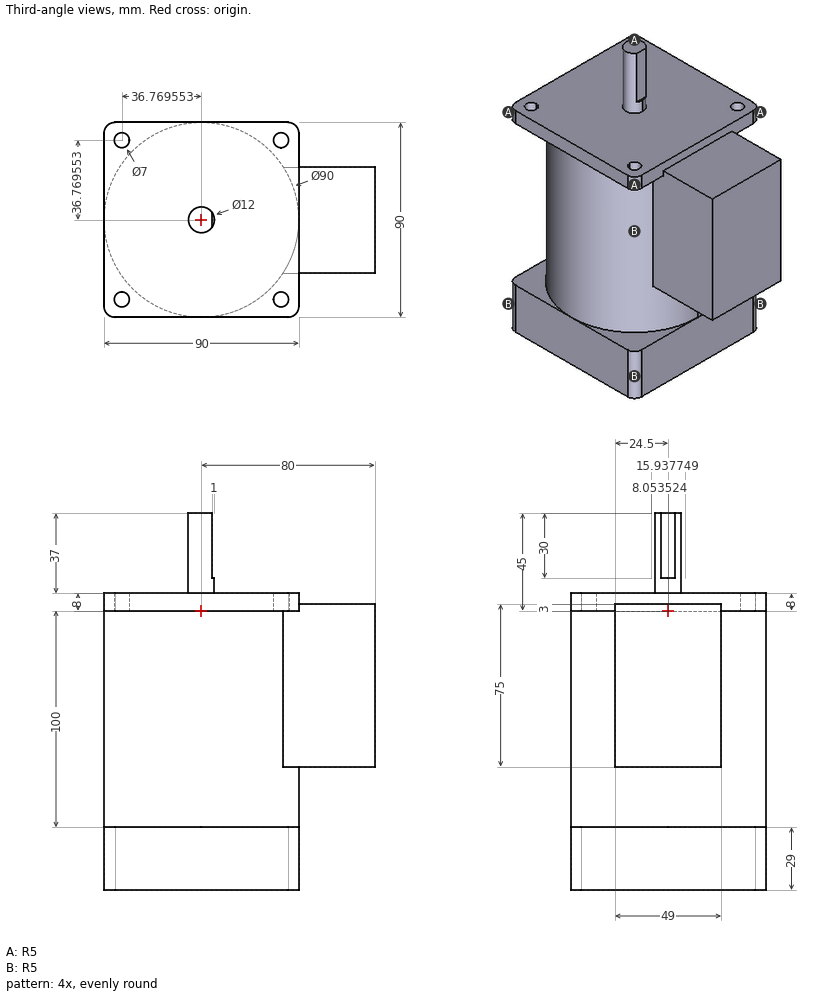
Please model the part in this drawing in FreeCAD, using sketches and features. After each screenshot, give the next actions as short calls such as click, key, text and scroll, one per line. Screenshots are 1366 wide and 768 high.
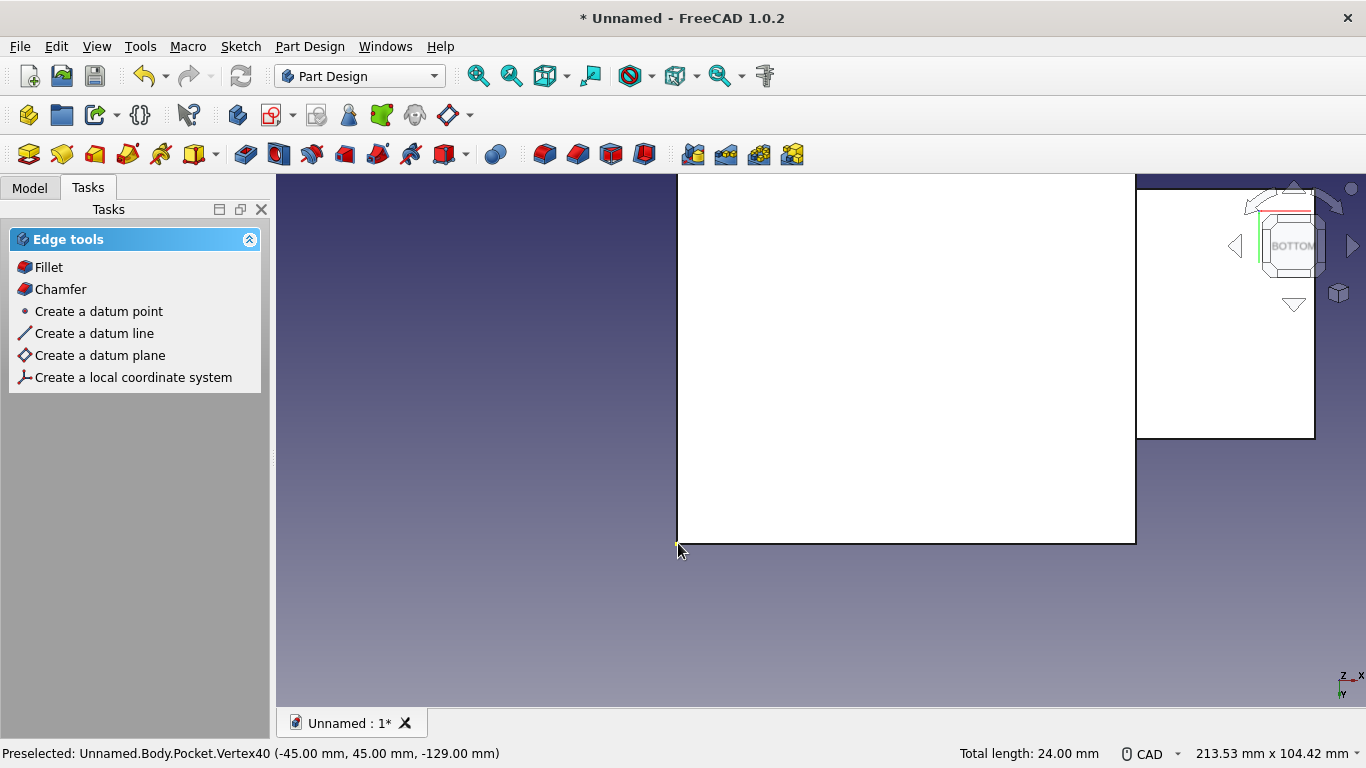
key(v)
key(f)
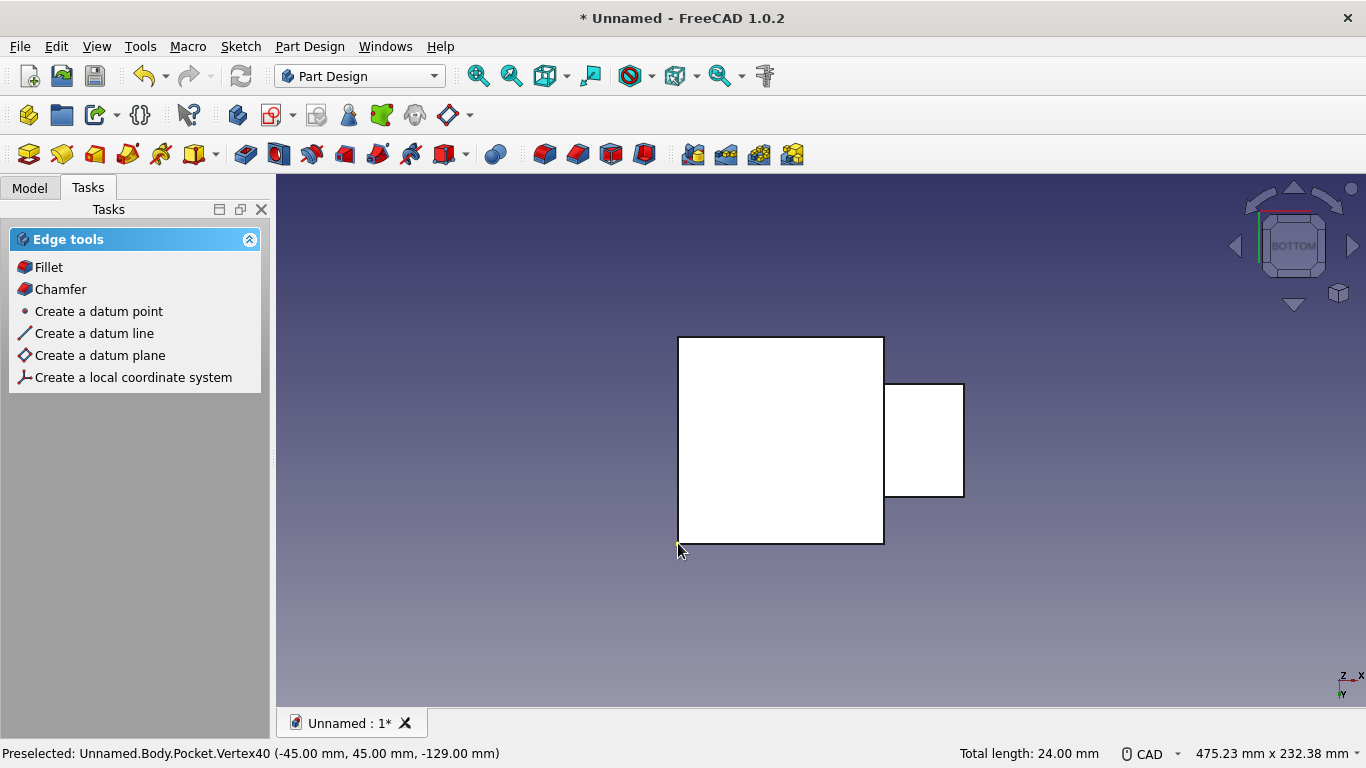
key(4)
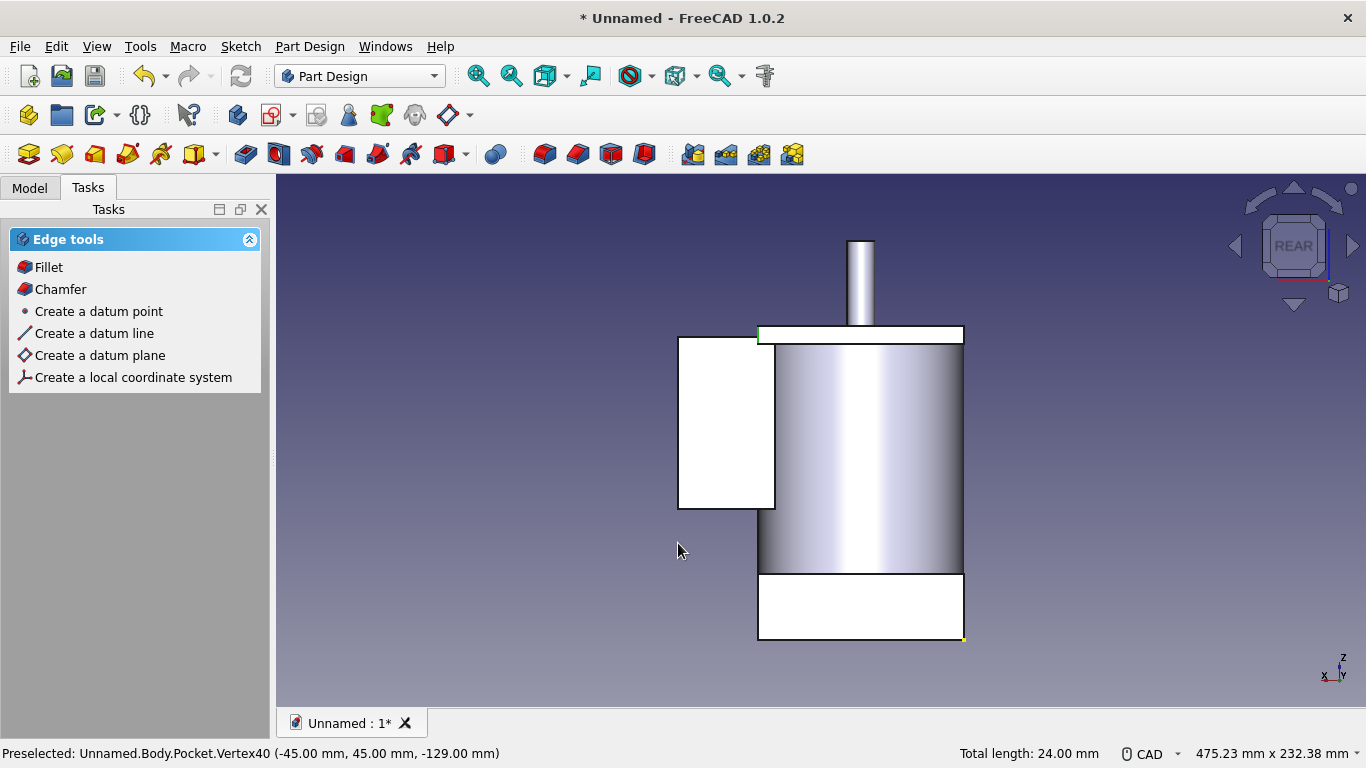
click(964, 334, ctrl)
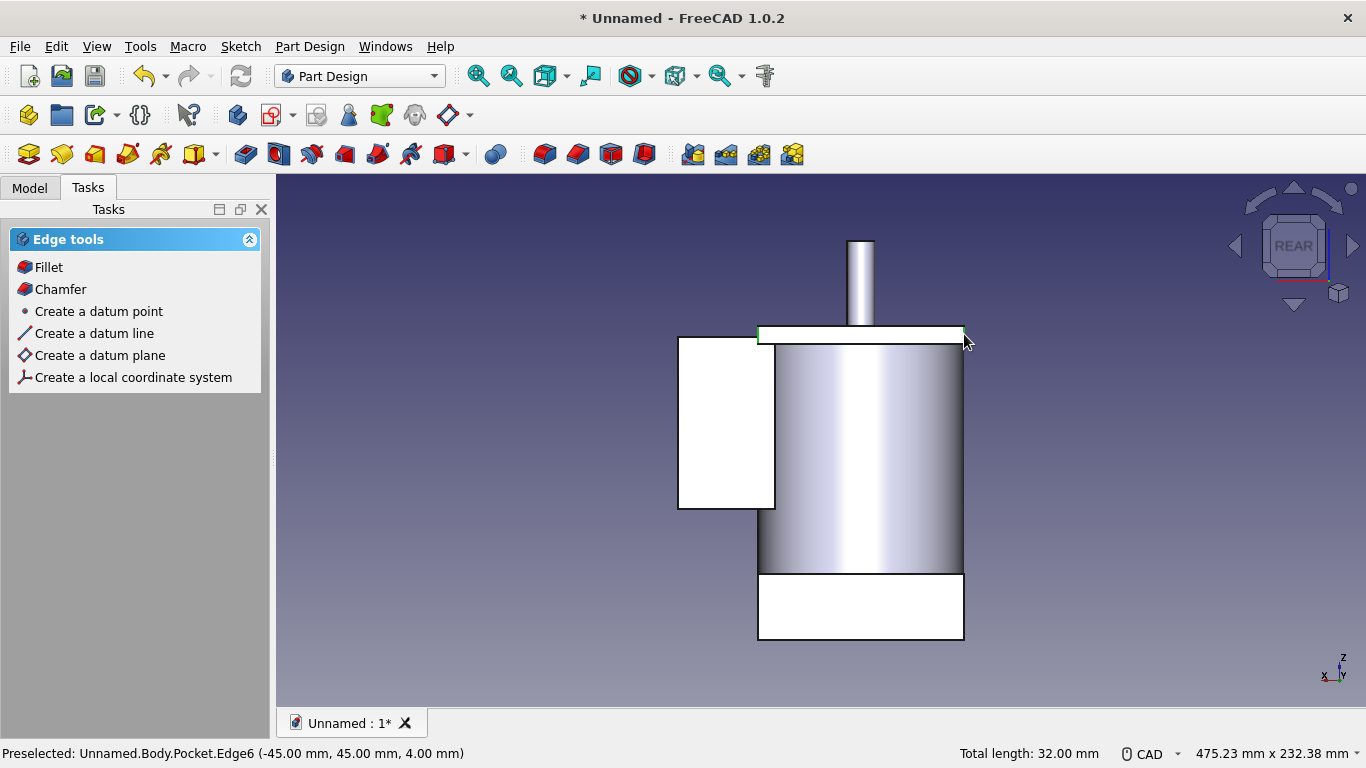
click(545, 154)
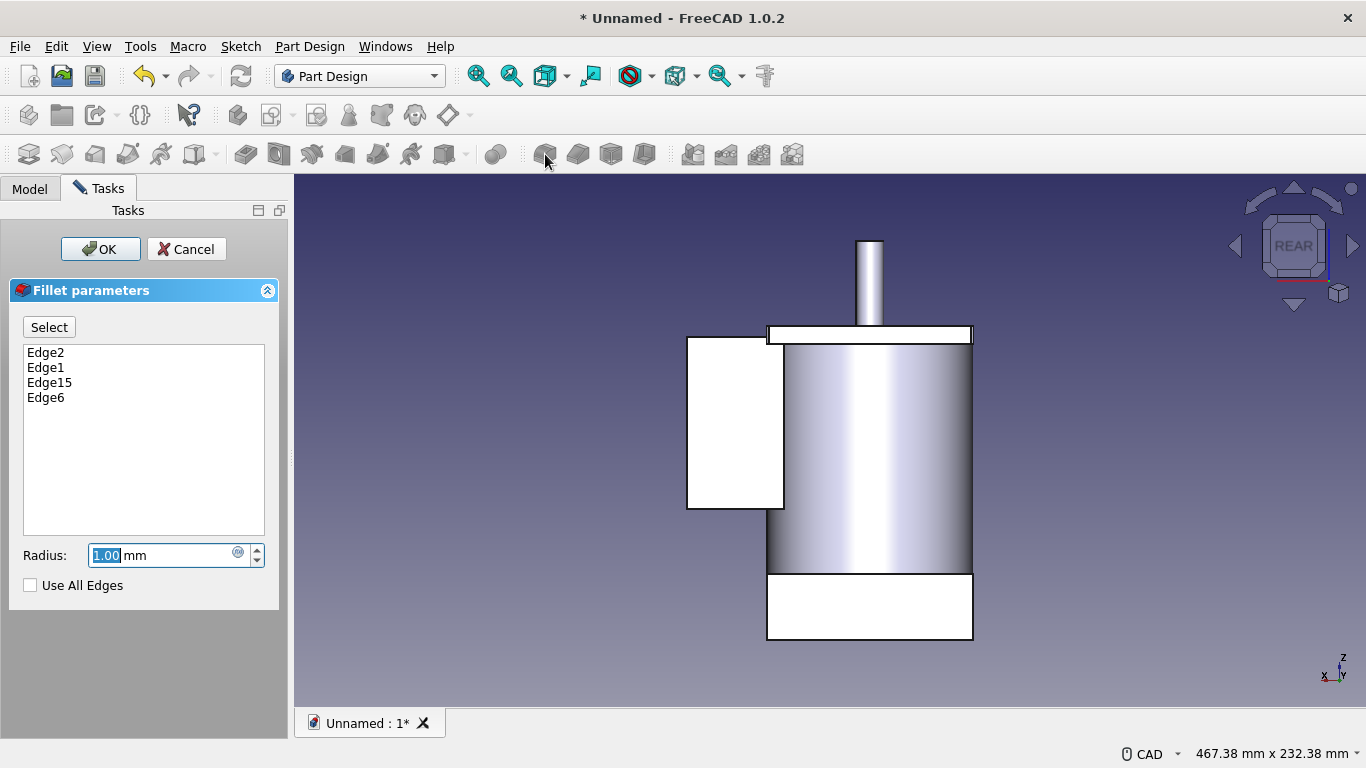
text(5)
key(Tab)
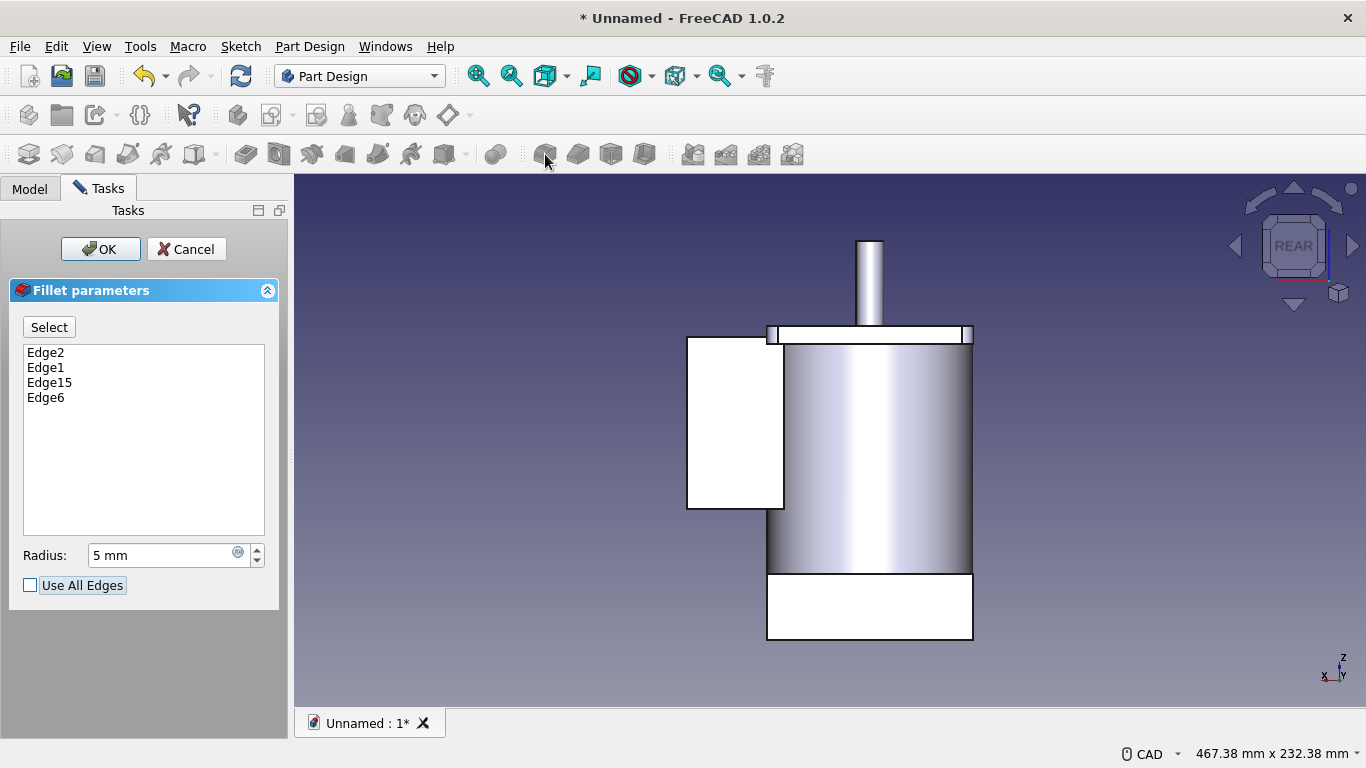
click(101, 249)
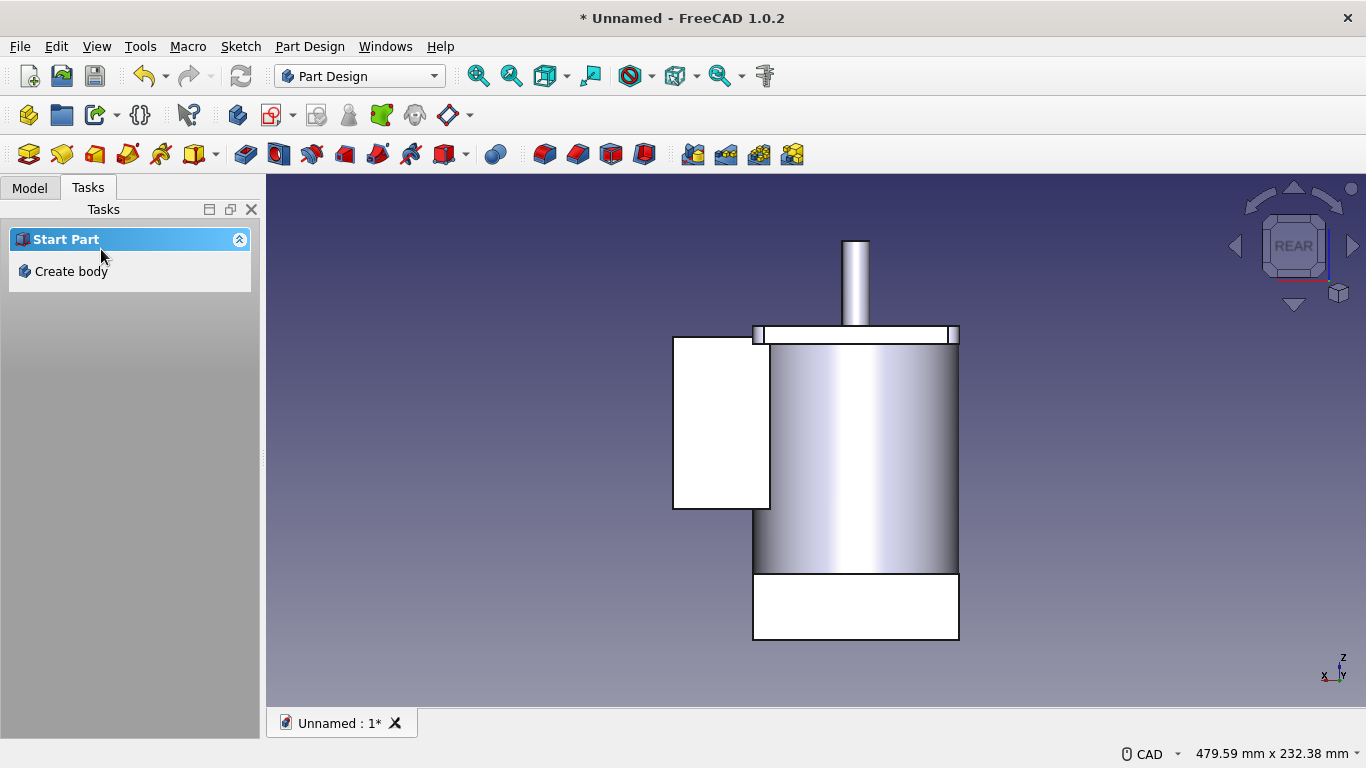
click(753, 606)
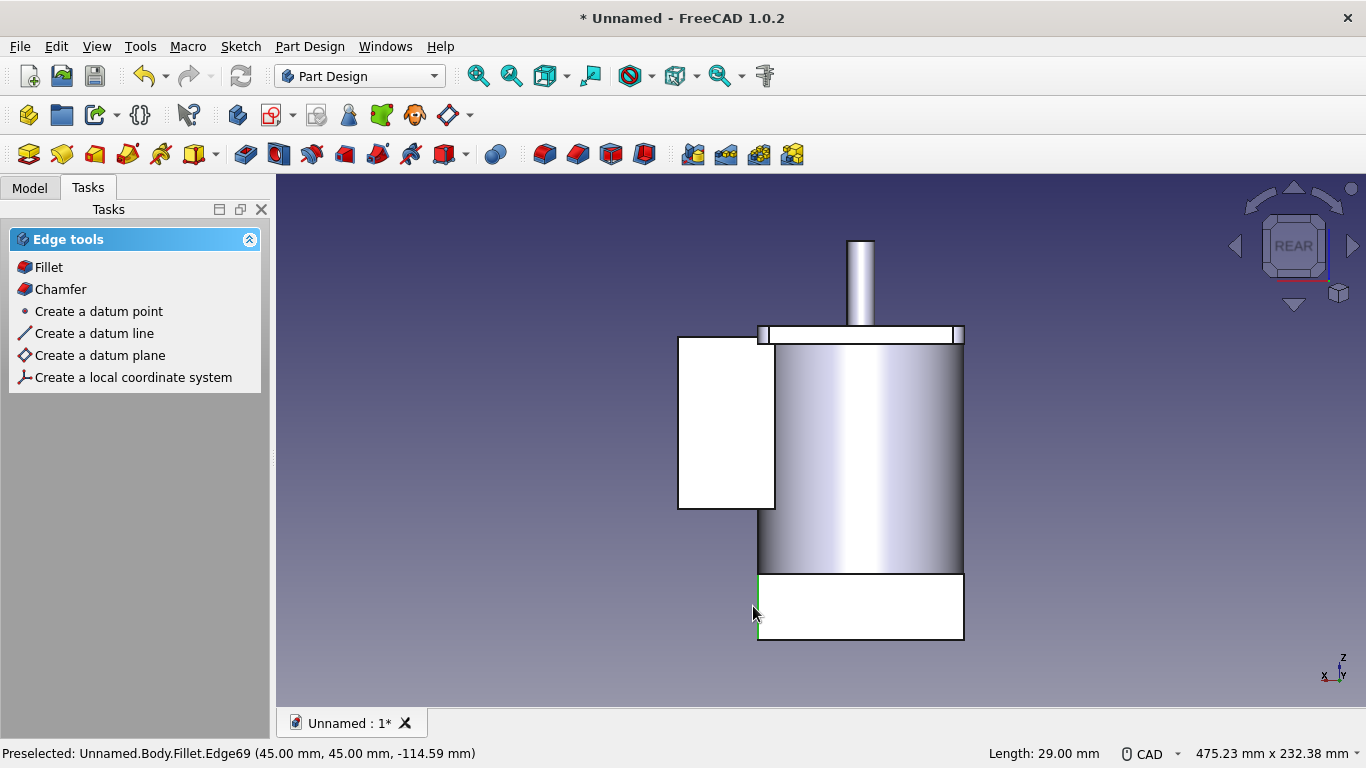
click(964, 606, ctrl)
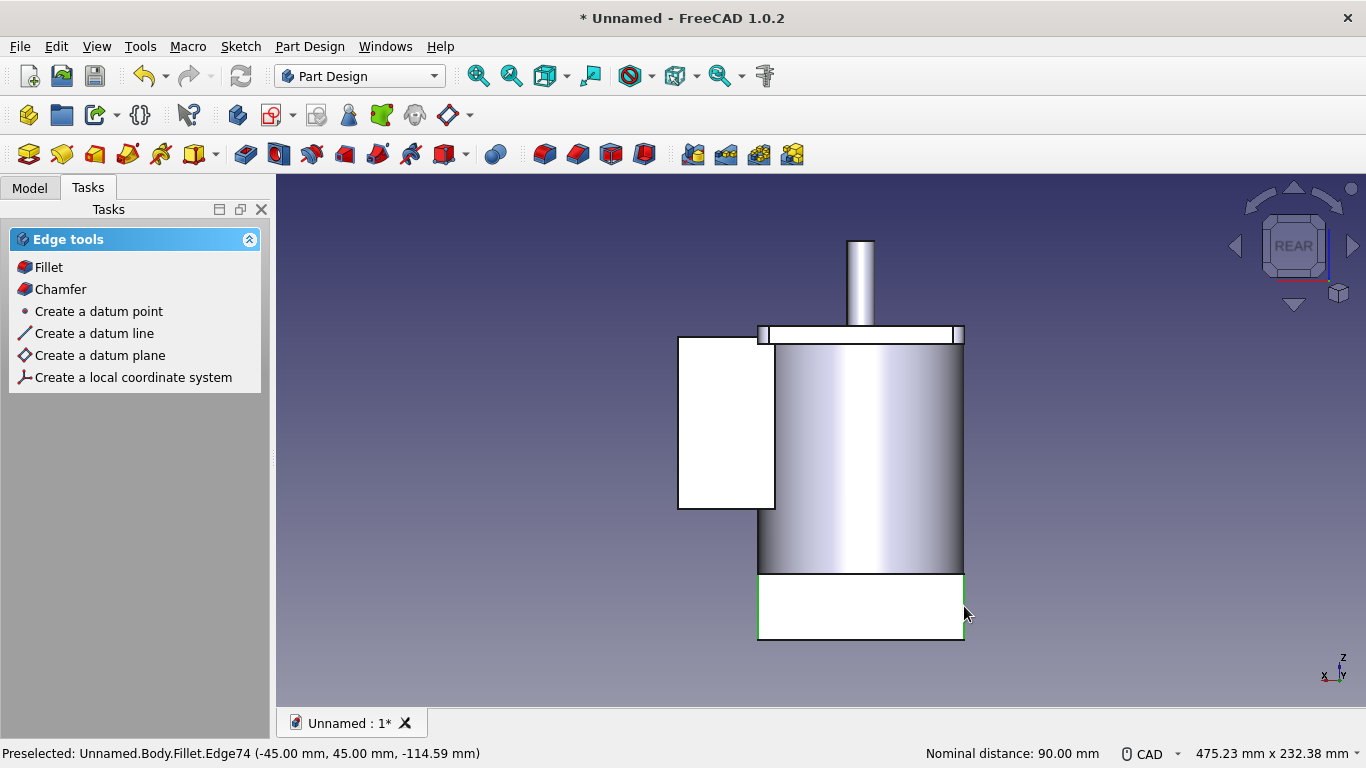
key(0)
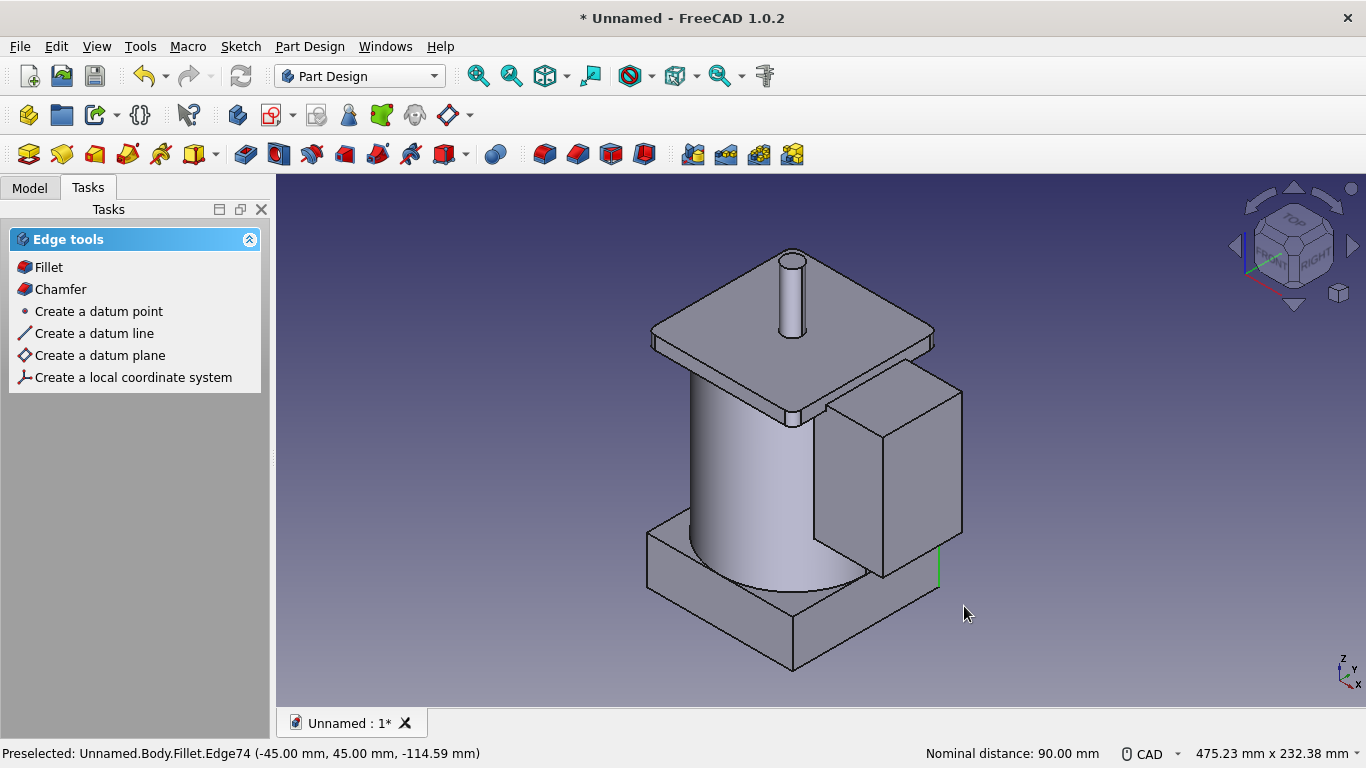
click(793, 643, ctrl)